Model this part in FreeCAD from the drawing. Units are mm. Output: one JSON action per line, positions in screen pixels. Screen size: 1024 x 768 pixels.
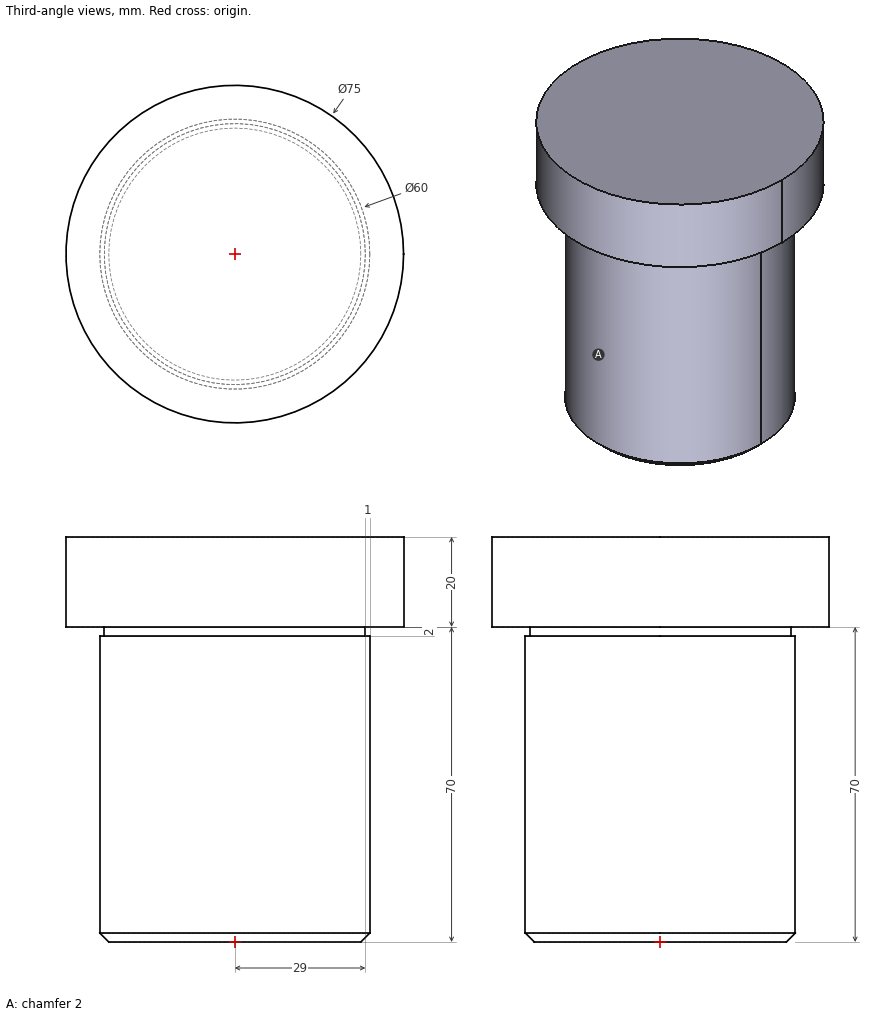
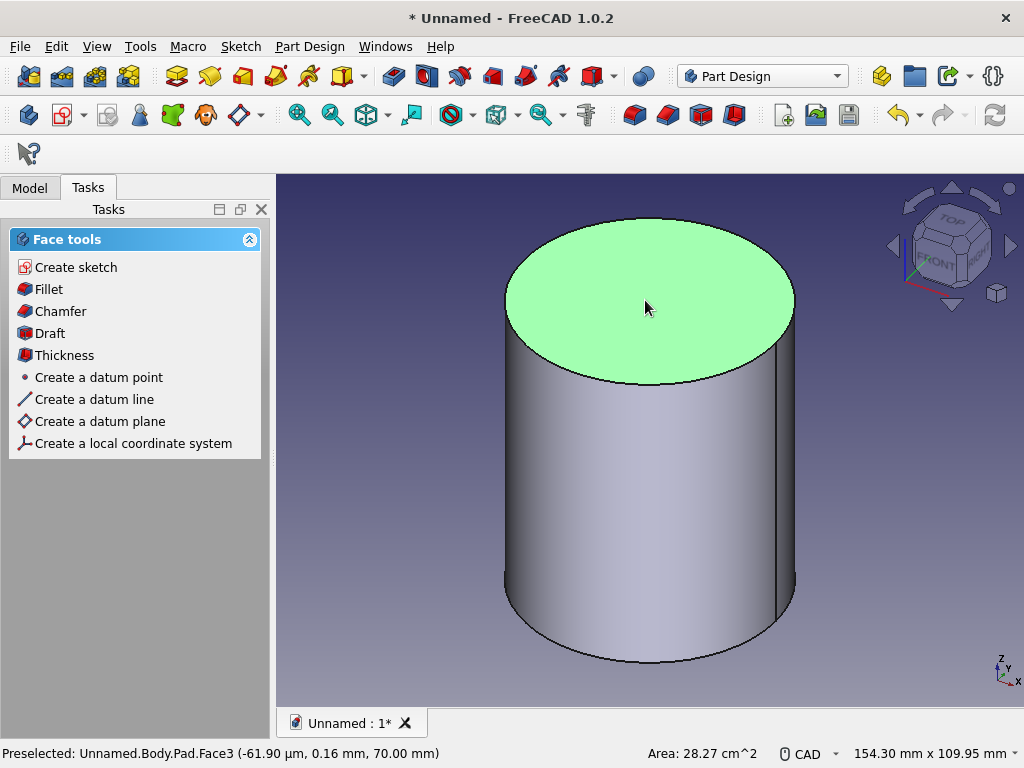
{"action": "left_click", "coordinate": [62, 116]}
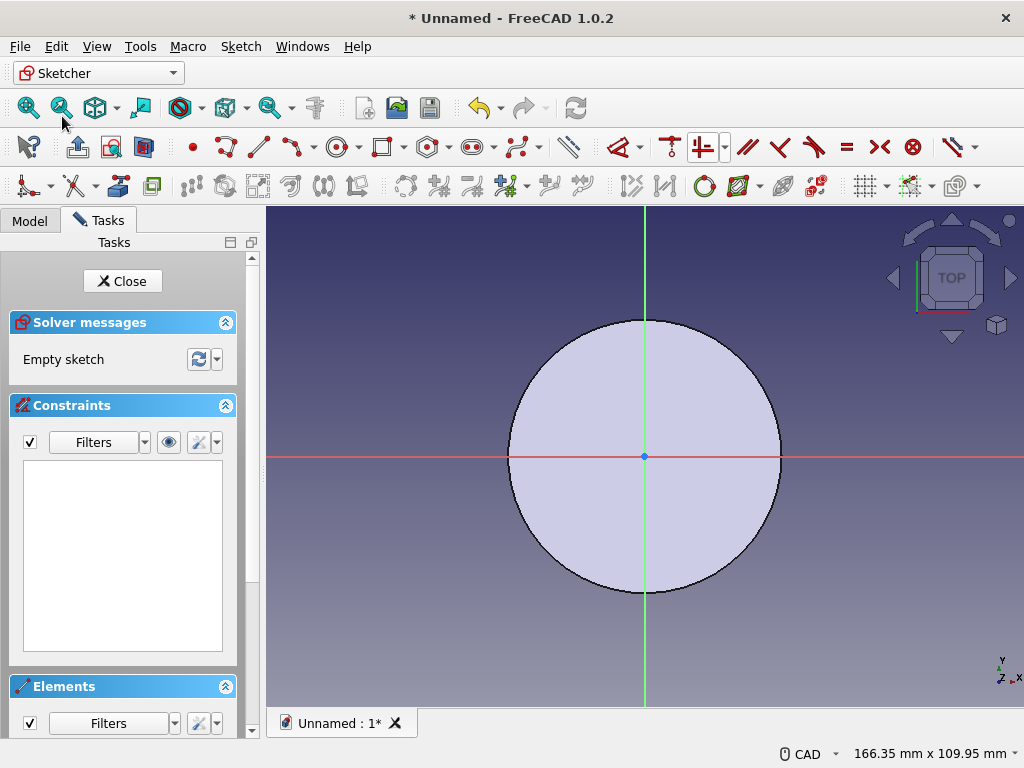
{"action": "left_click", "coordinate": [336, 148]}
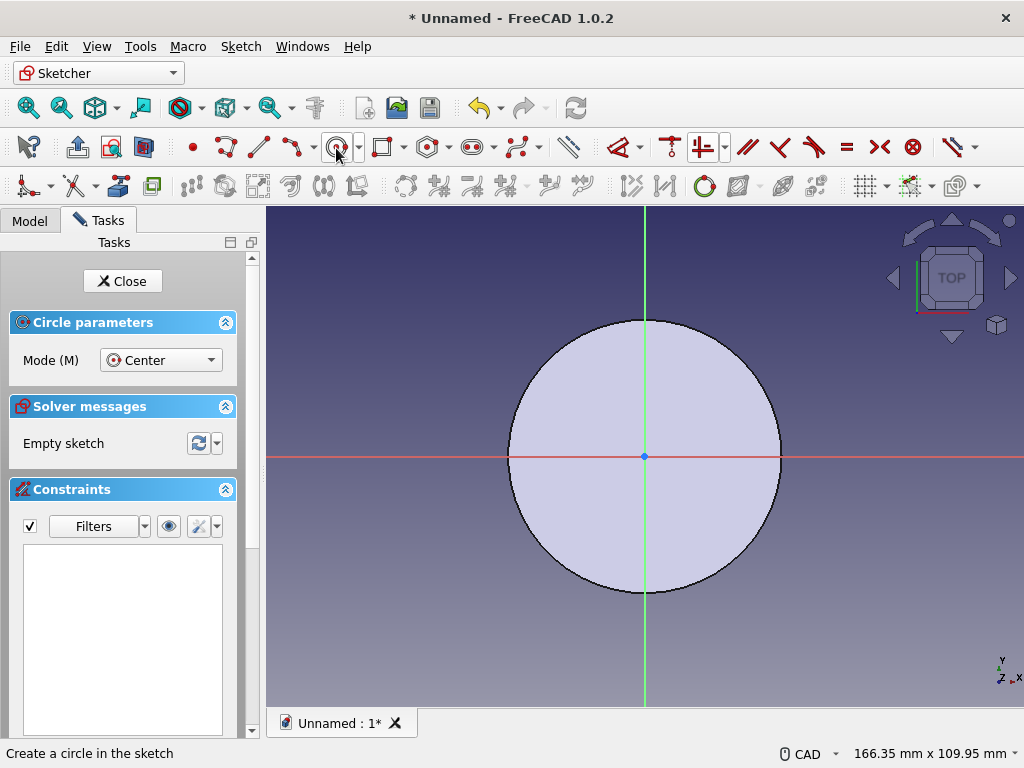
{"action": "left_click", "coordinate": [645, 456]}
{"action": "mouse_move", "coordinate": [766, 336]}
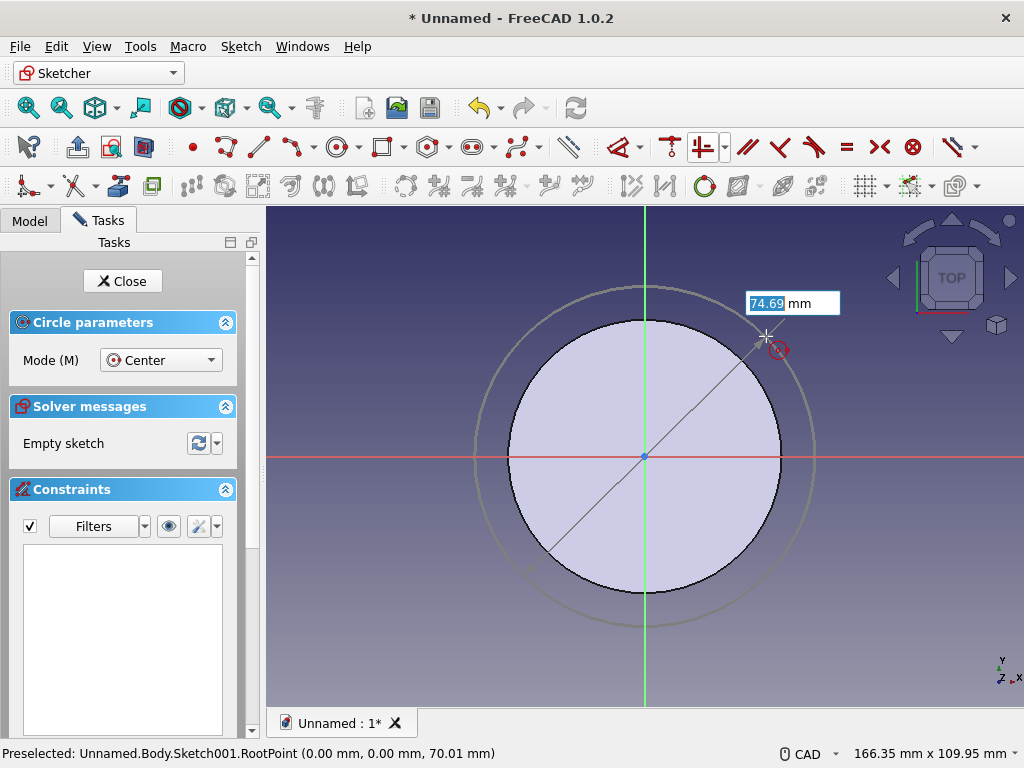
{"action": "type", "text": "75"}
{"action": "key", "text": "Return"}
{"action": "key", "text": "Escape"}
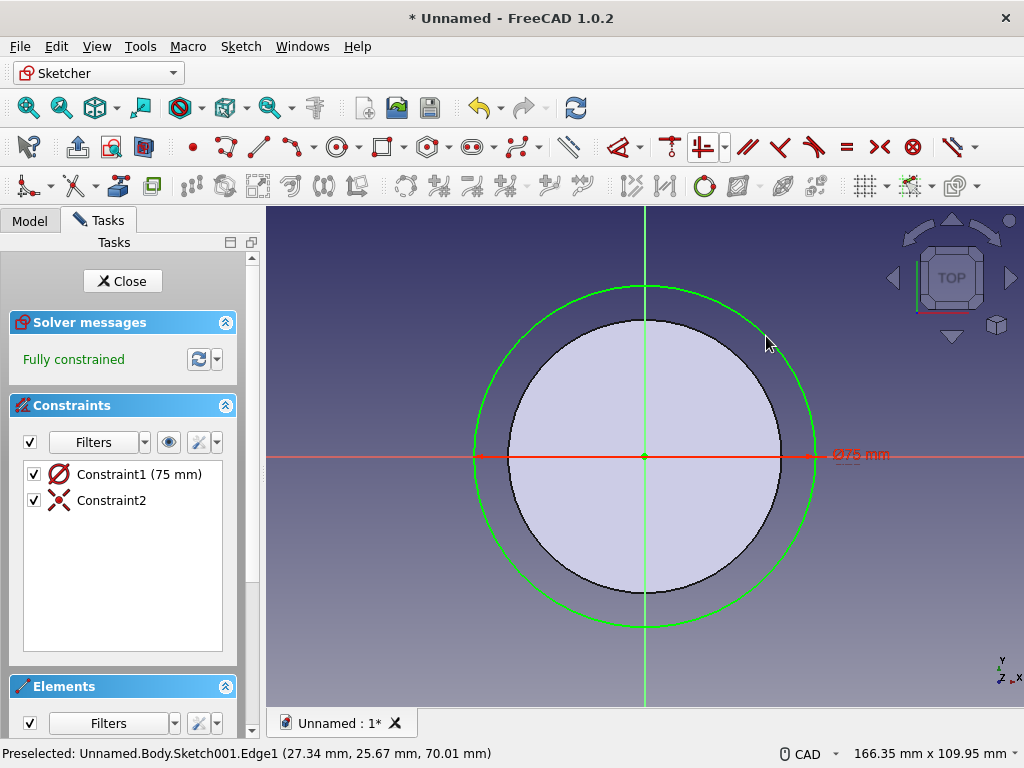
{"action": "left_click", "coordinate": [123, 281]}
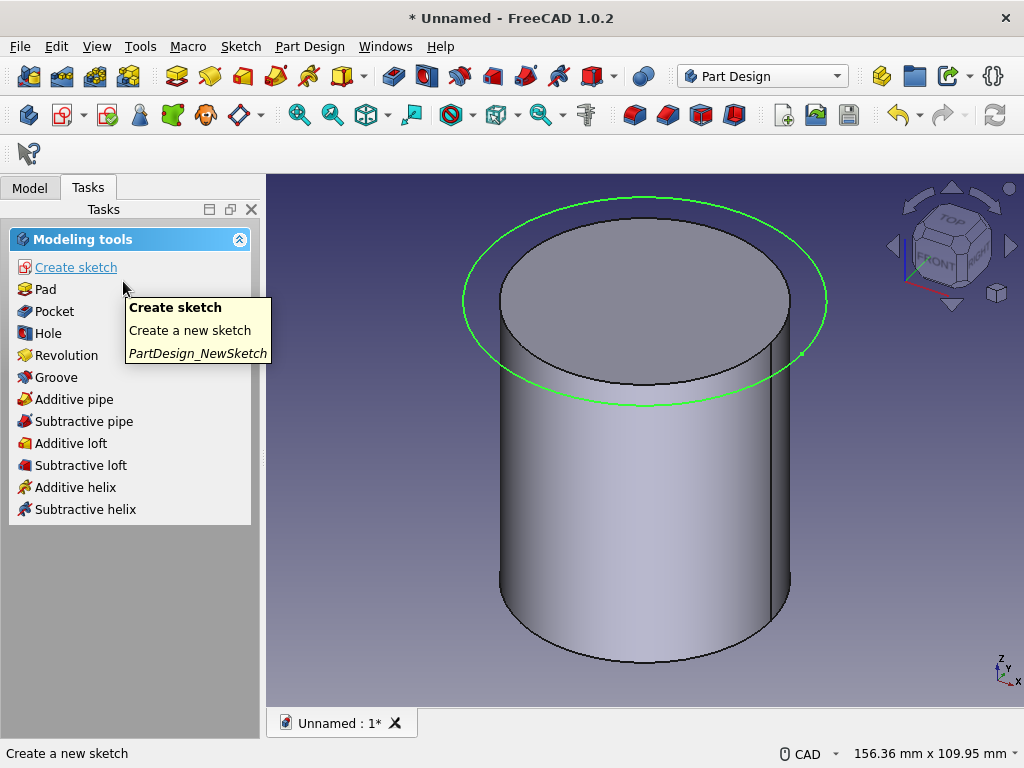
{"action": "left_click", "coordinate": [177, 76]}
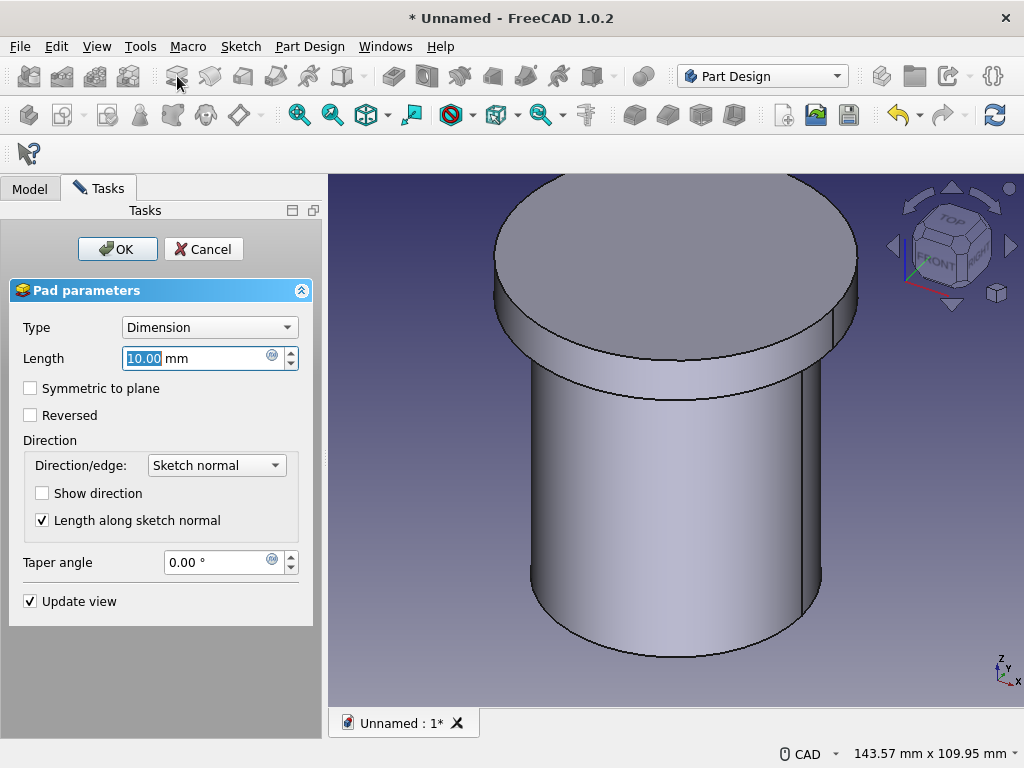
{"action": "type", "text": "20"}
{"action": "key", "text": "Tab"}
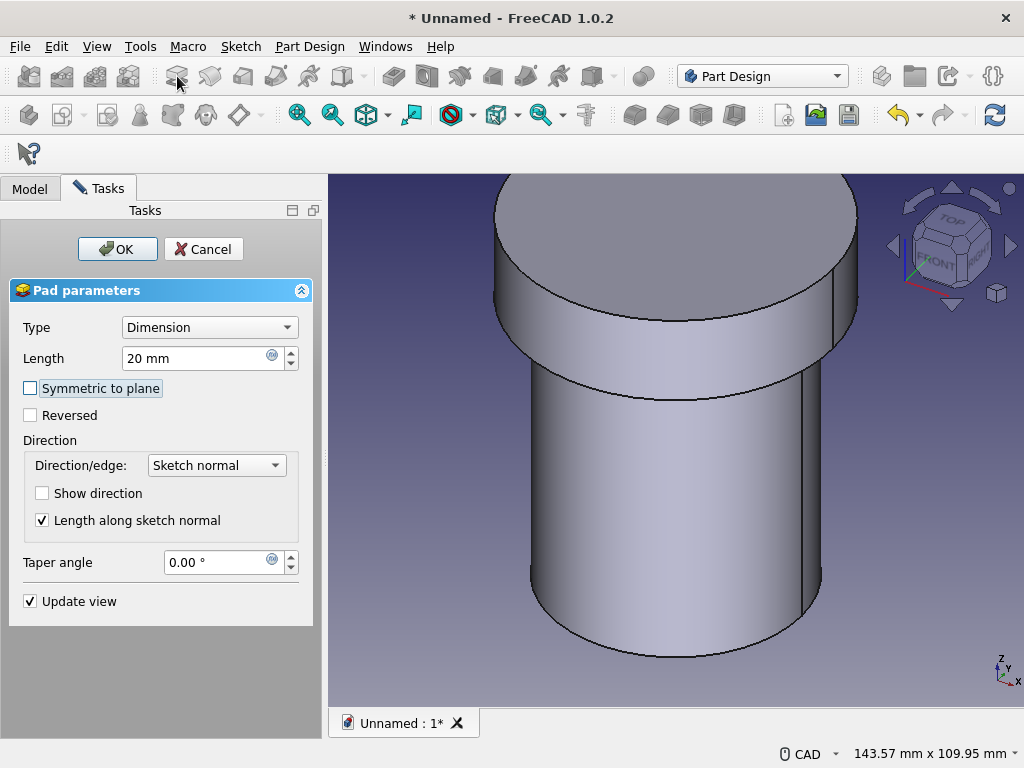
{"action": "left_click", "coordinate": [118, 249]}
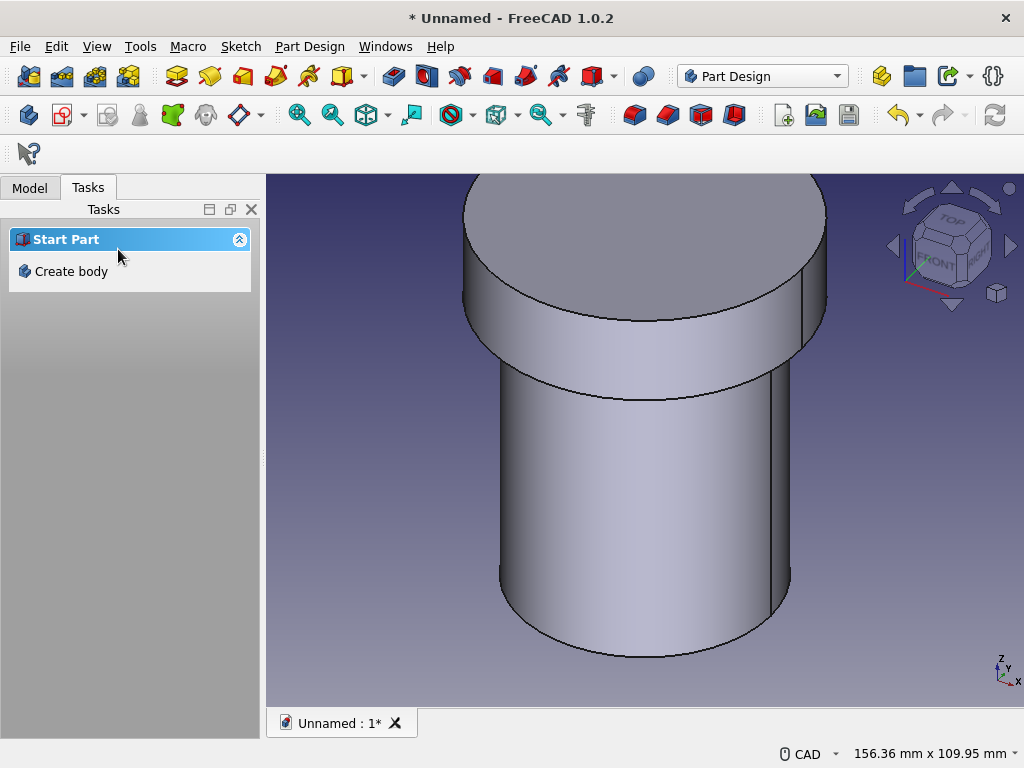
{"action": "key", "text": "v f"}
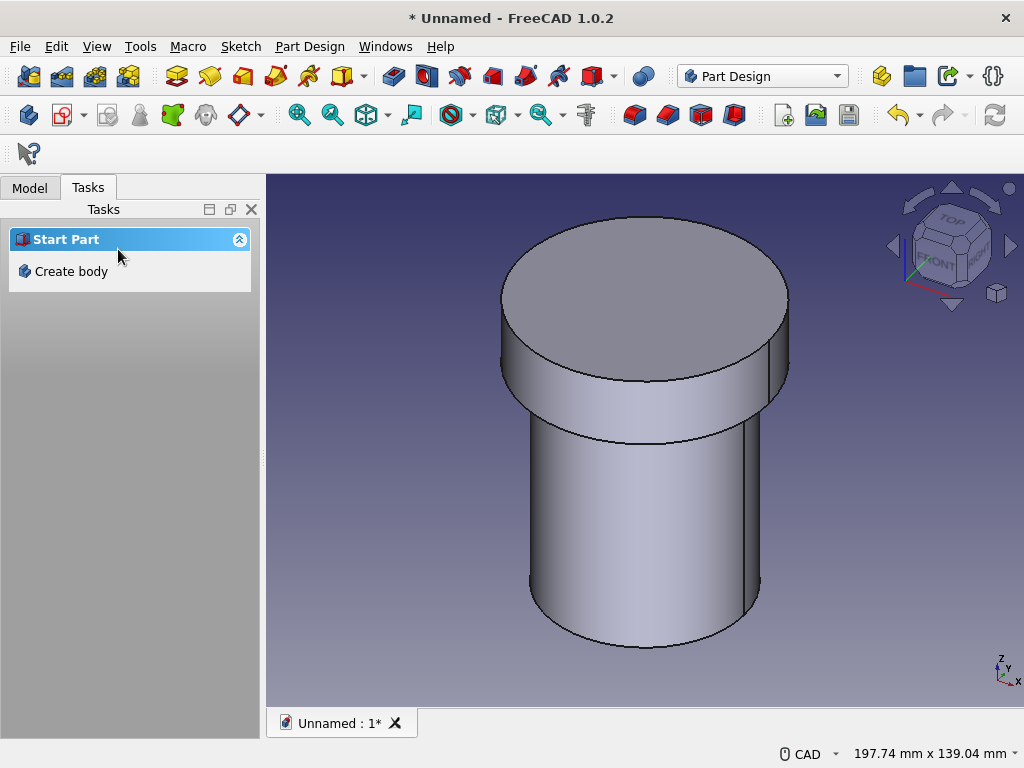
{"action": "left_click", "coordinate": [559, 625]}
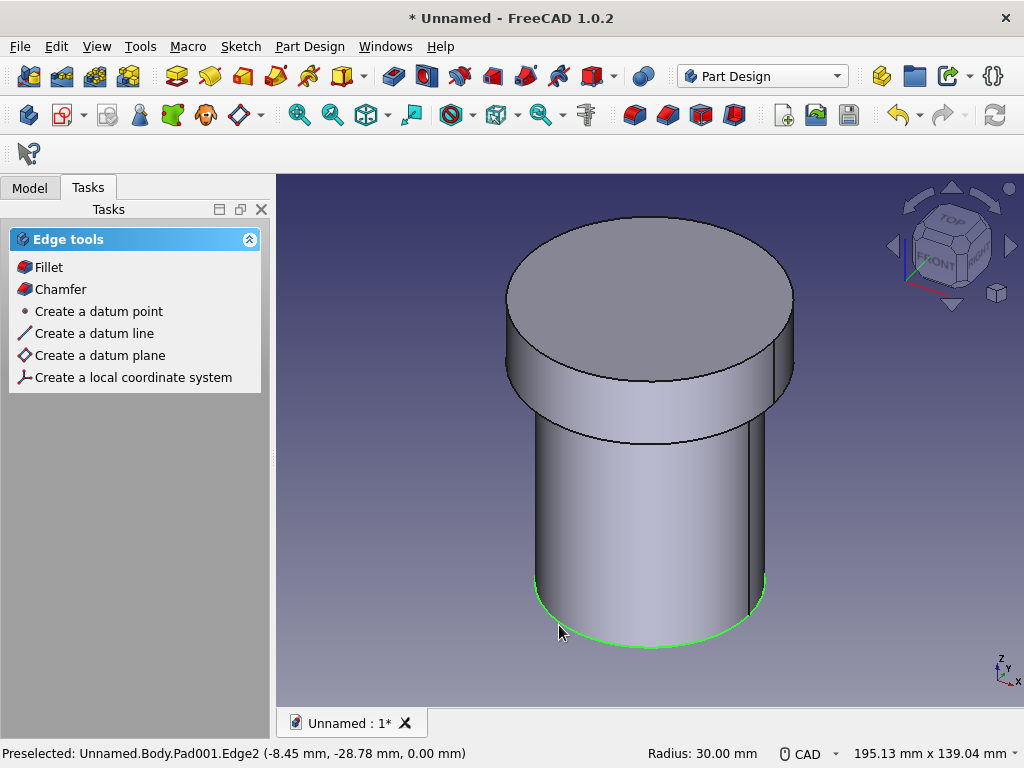
{"action": "left_click", "coordinate": [668, 116]}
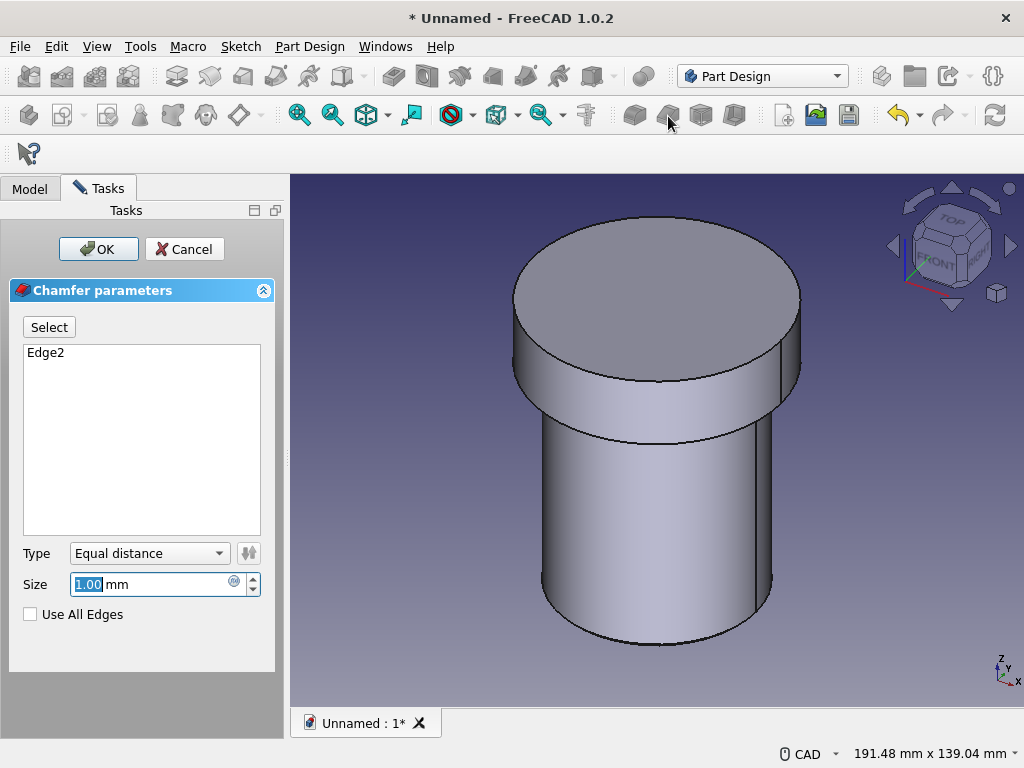
{"action": "type", "text": "2"}
{"action": "key", "text": "Tab"}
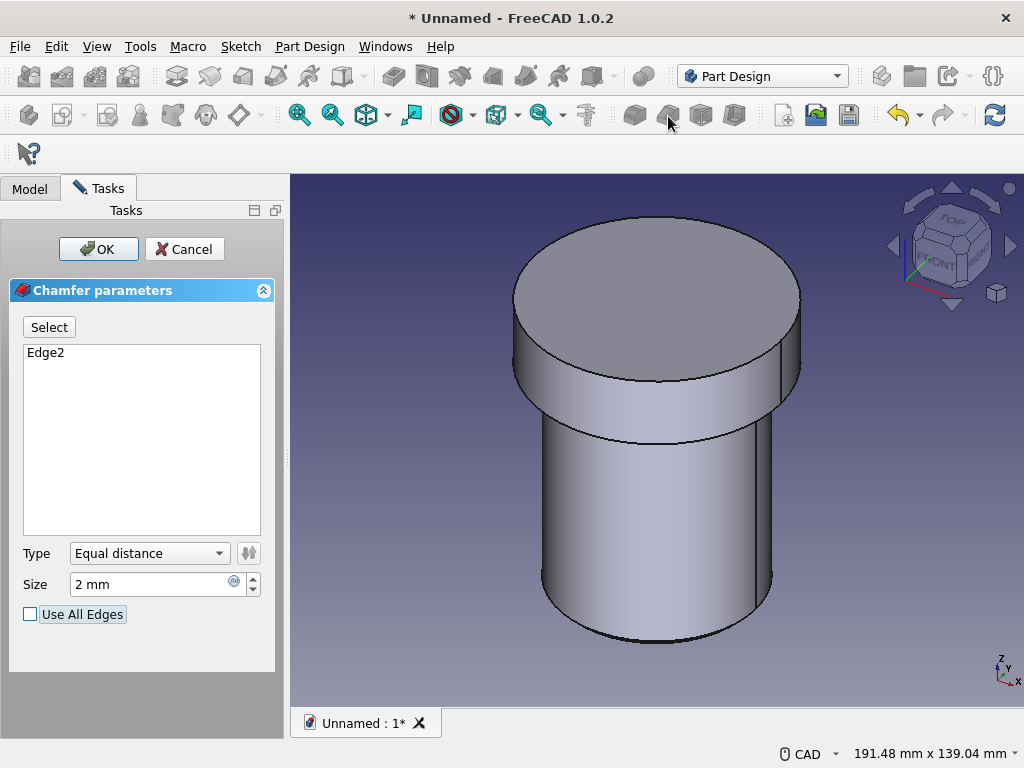
{"action": "left_click", "coordinate": [99, 249]}